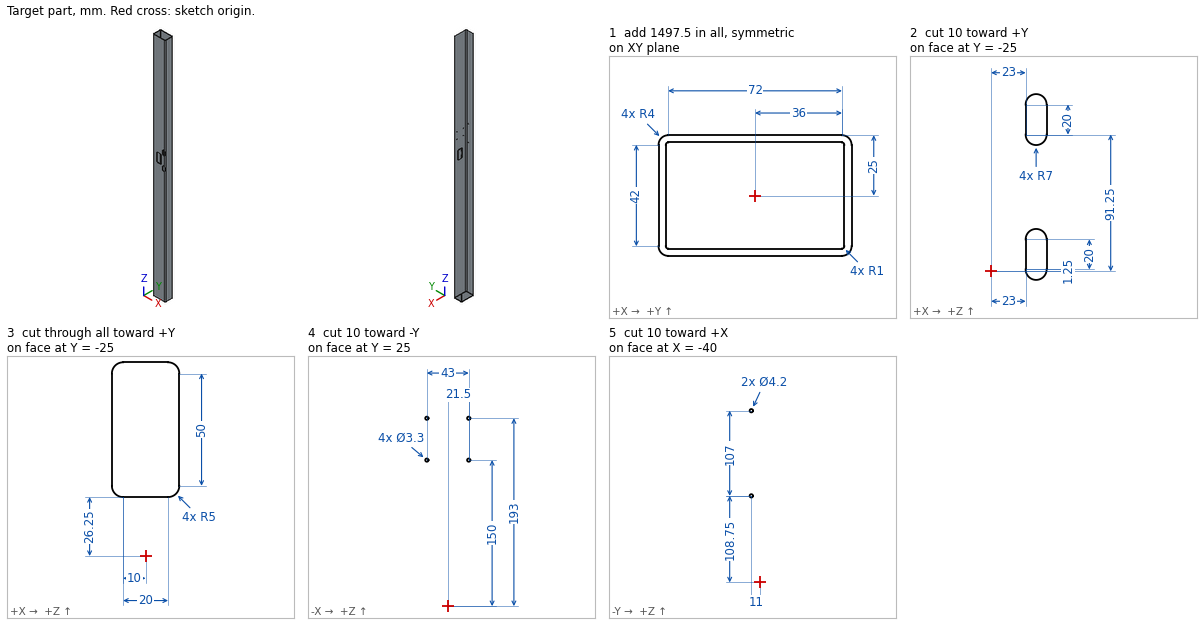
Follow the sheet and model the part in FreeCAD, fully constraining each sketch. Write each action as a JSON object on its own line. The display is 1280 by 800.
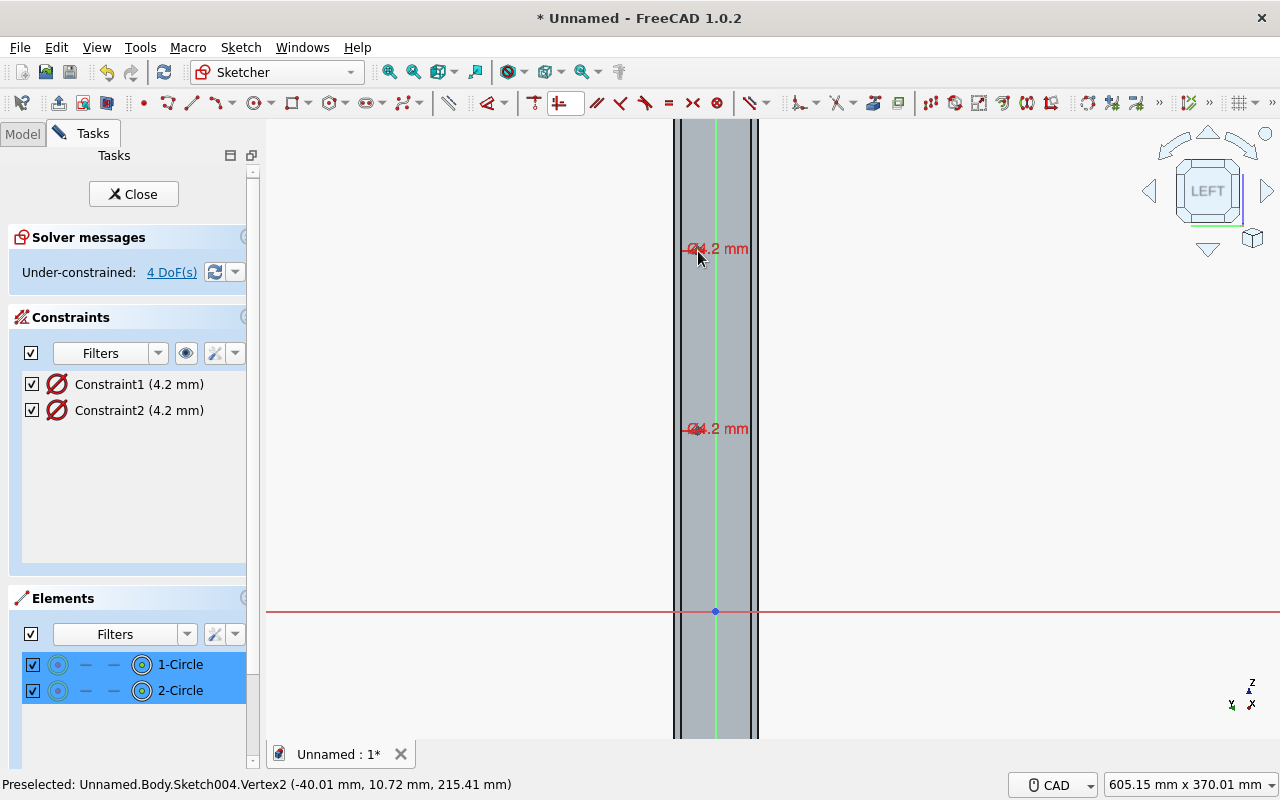
{"action": "key", "text": "v"}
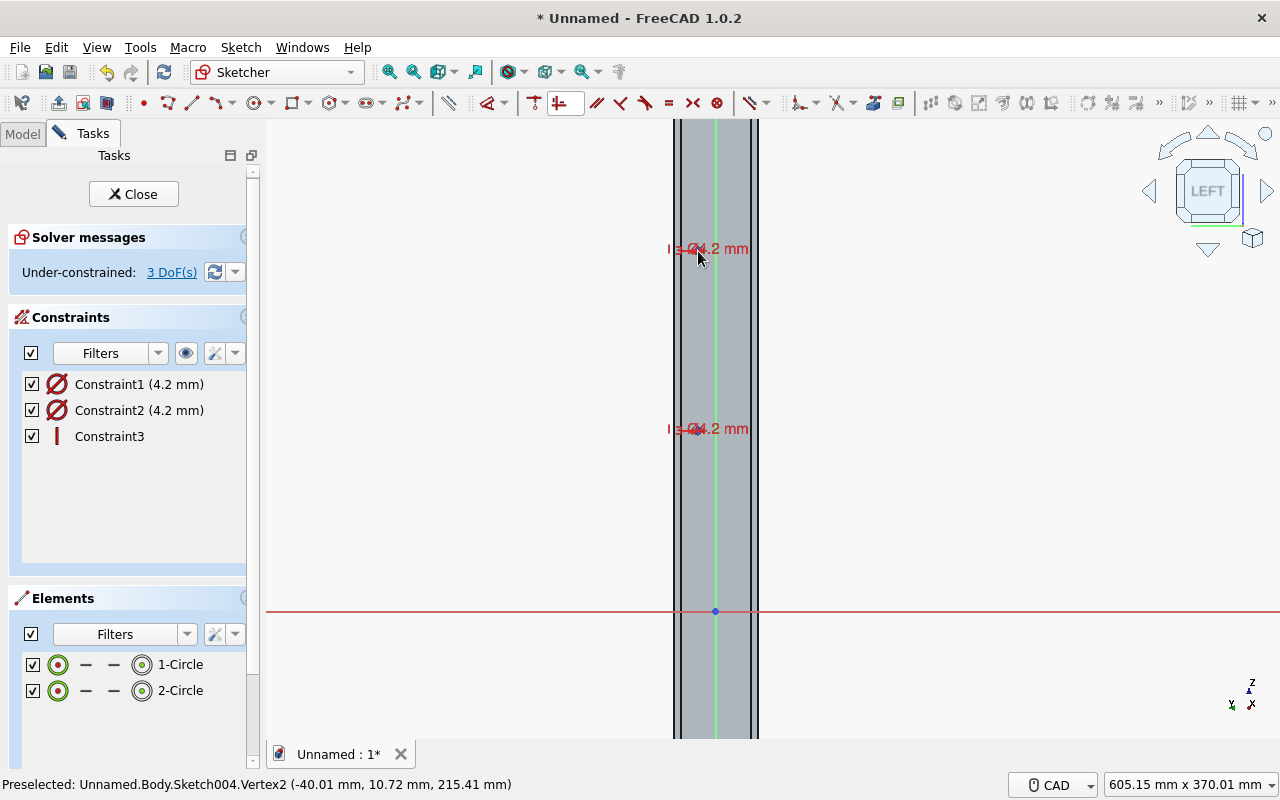
{"action": "left_click", "coordinate": [488, 104]}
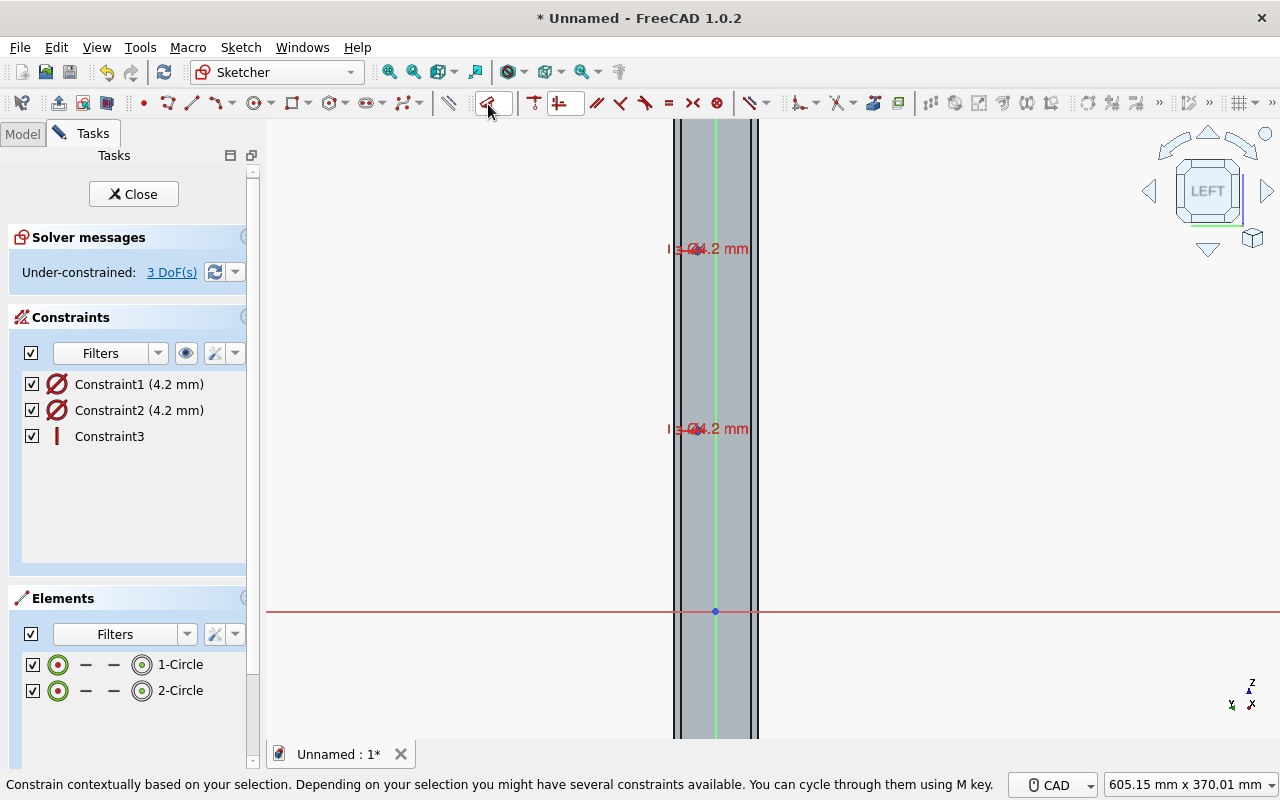
{"action": "scroll", "coordinate": [698, 431], "scroll_direction": "up", "scroll_amount": 4}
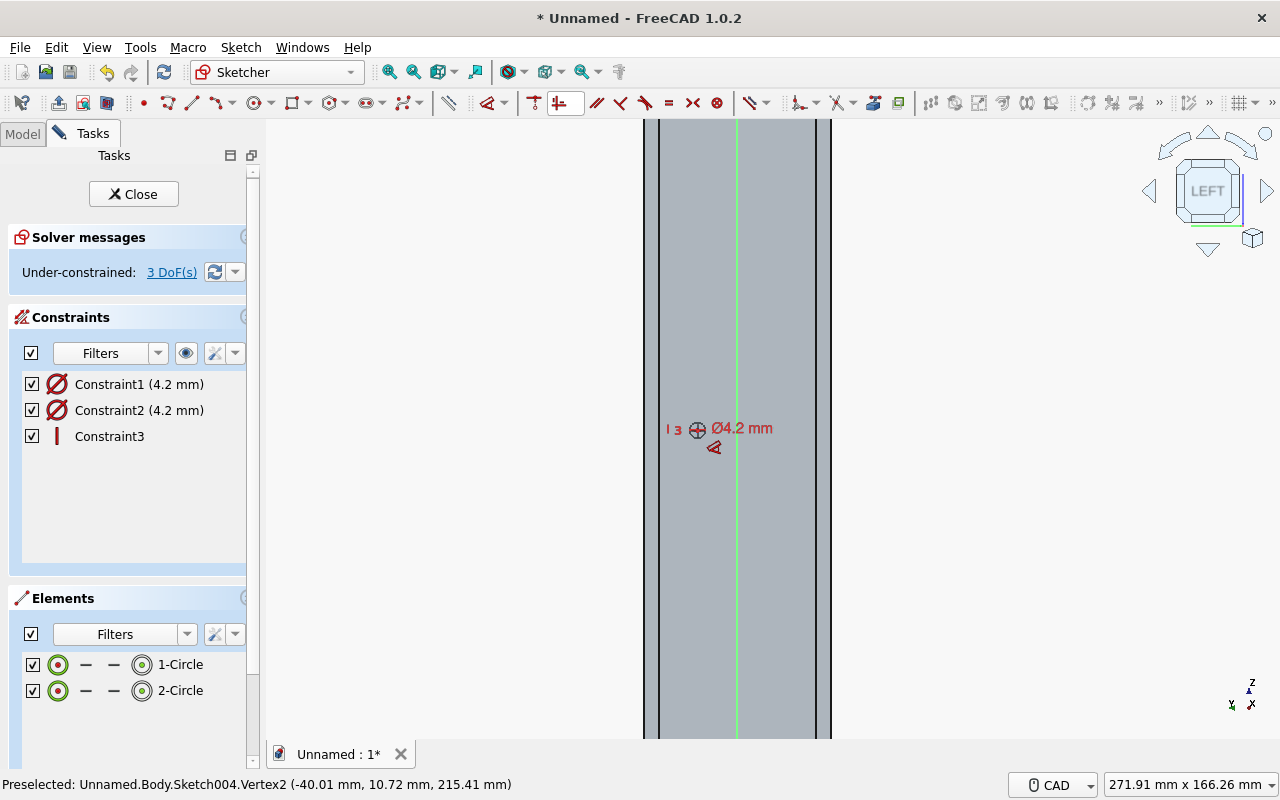
{"action": "left_click", "coordinate": [697, 430]}
{"action": "left_click", "coordinate": [717, 396]}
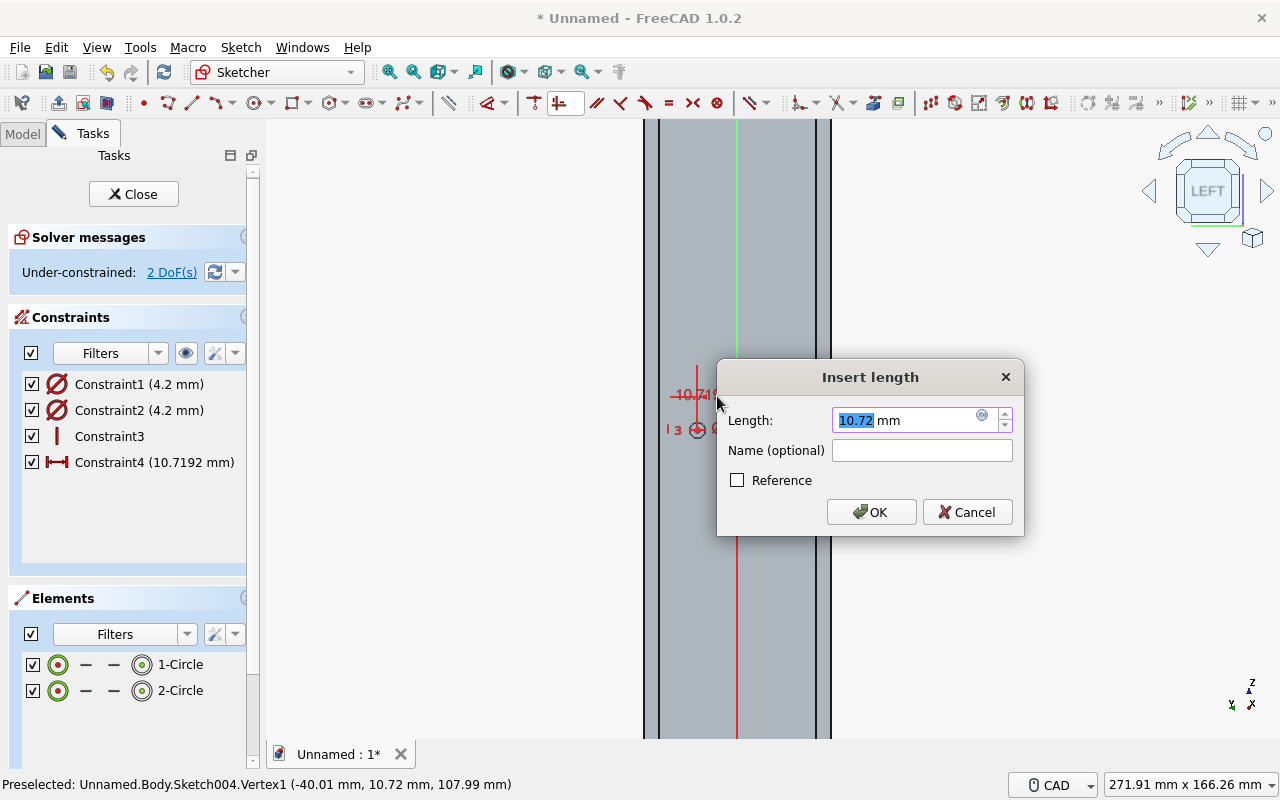
{"action": "type", "text": "11"}
{"action": "key", "text": "Return"}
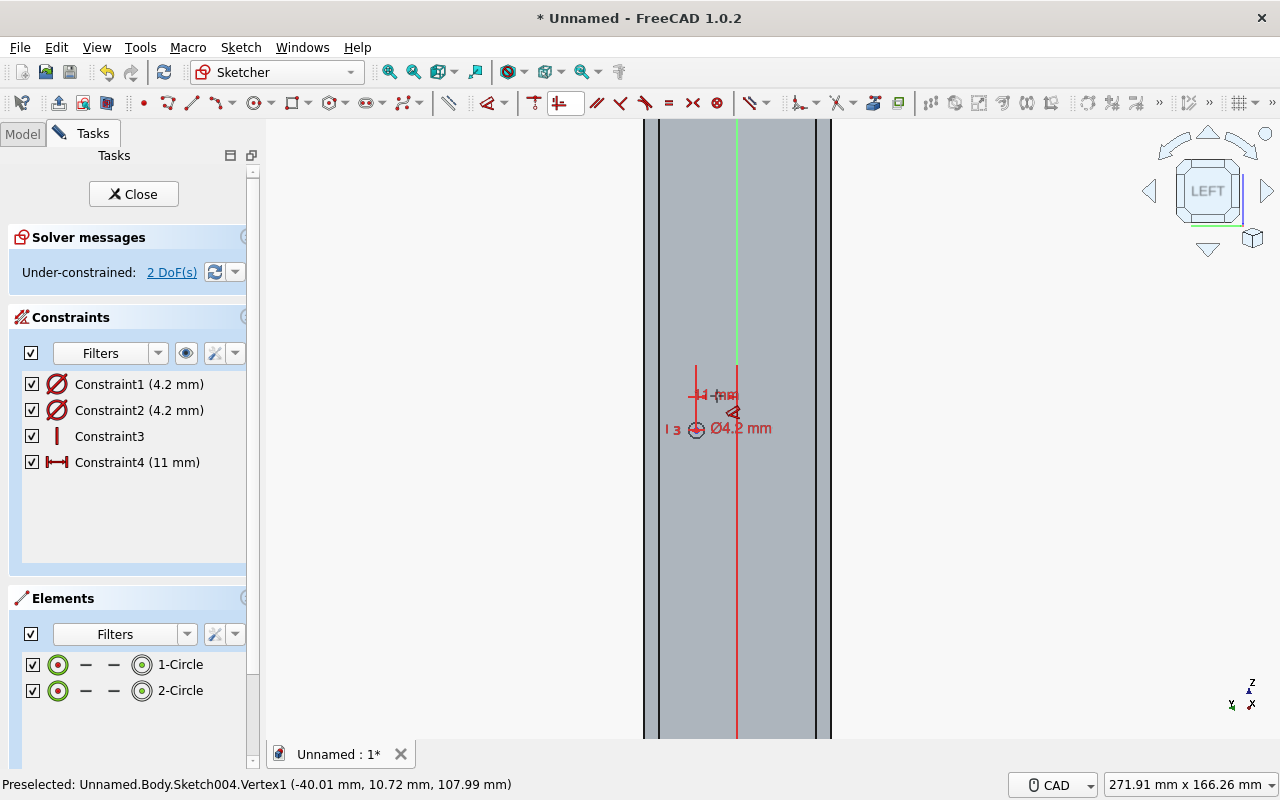
{"action": "left_click", "coordinate": [696, 430]}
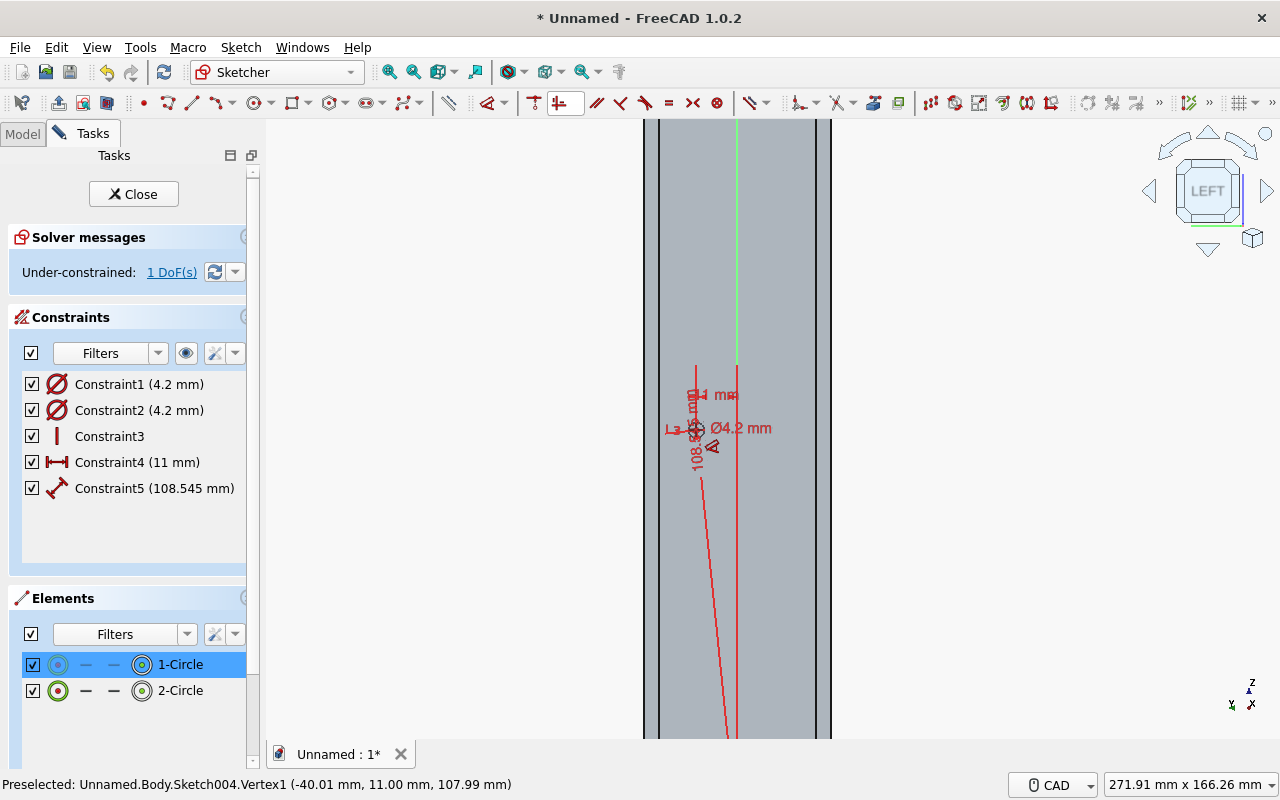
{"action": "scroll", "coordinate": [698, 431], "scroll_direction": "down", "scroll_amount": 4}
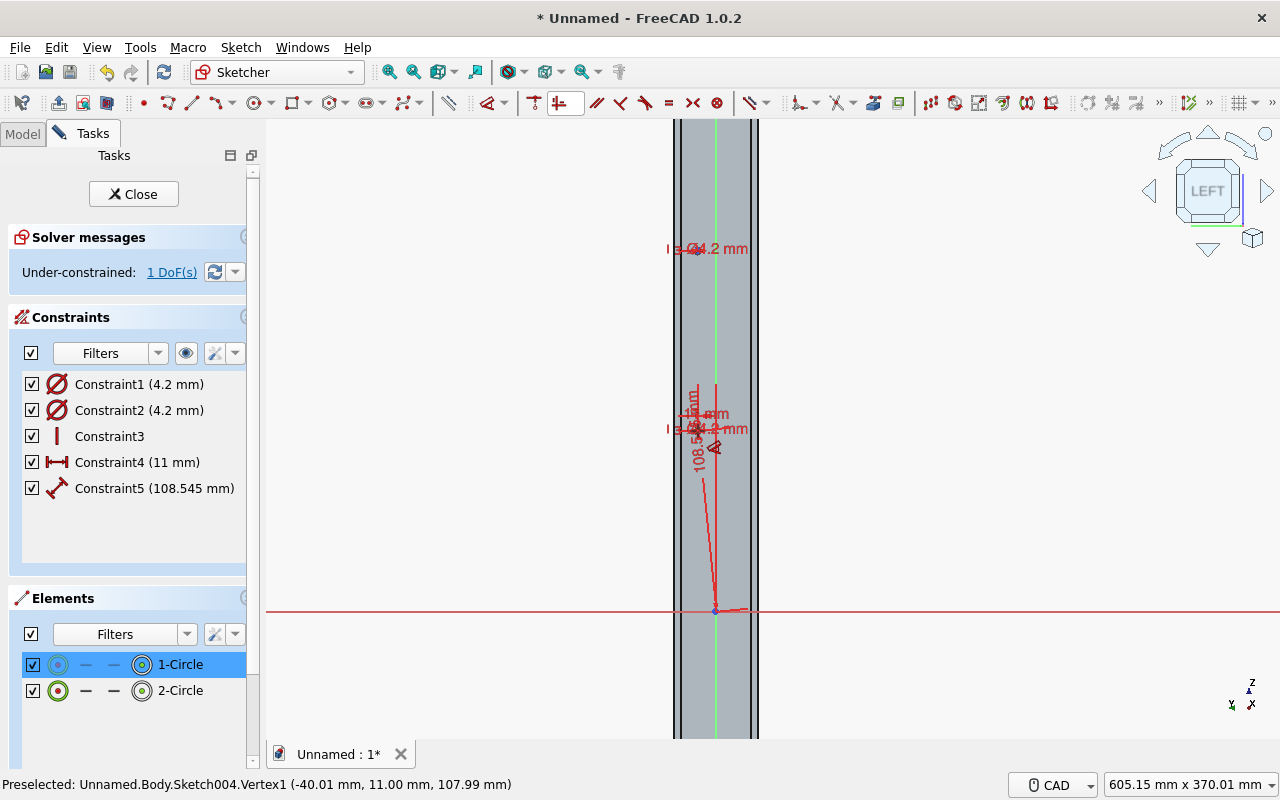
{"action": "left_click", "coordinate": [698, 251]}
{"action": "left_click", "coordinate": [664, 341]}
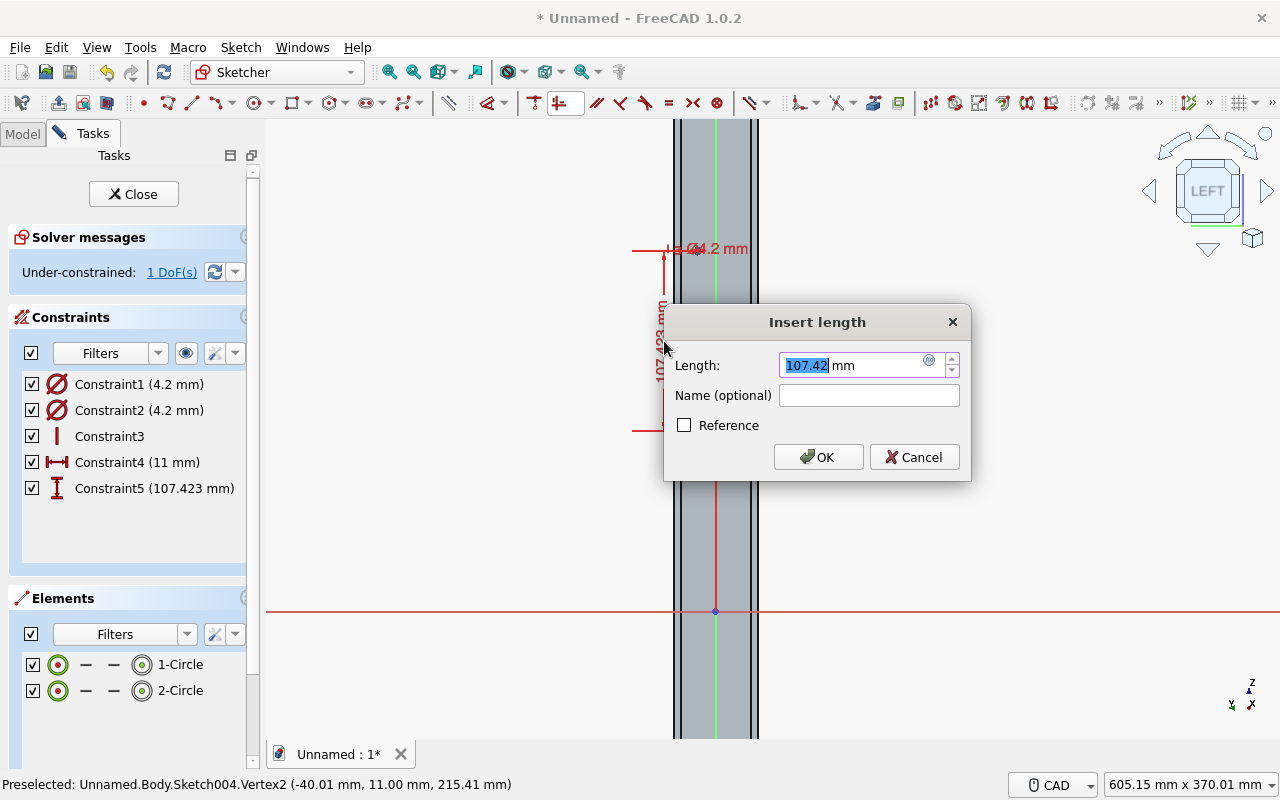
{"action": "type", "text": "107"}
{"action": "key", "text": "Return"}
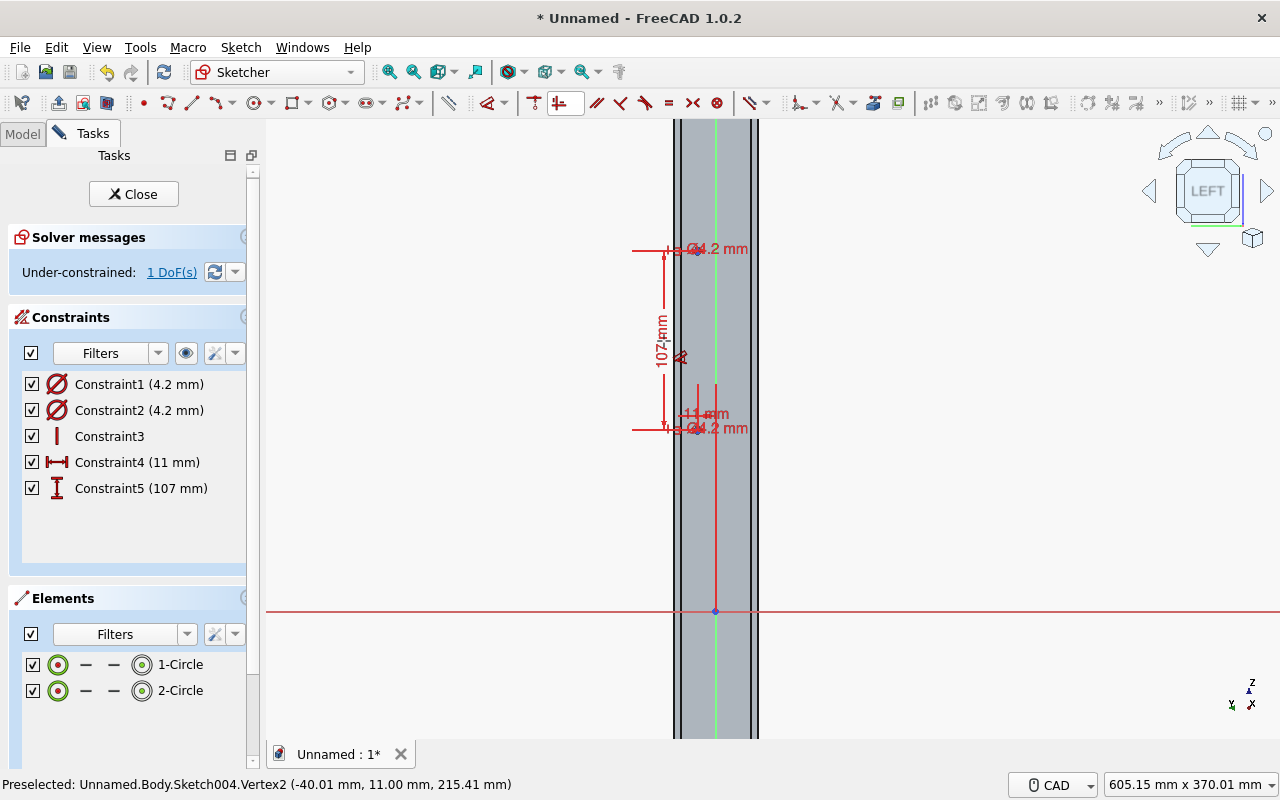
{"action": "left_click", "coordinate": [698, 430]}
{"action": "left_click", "coordinate": [750, 521]}